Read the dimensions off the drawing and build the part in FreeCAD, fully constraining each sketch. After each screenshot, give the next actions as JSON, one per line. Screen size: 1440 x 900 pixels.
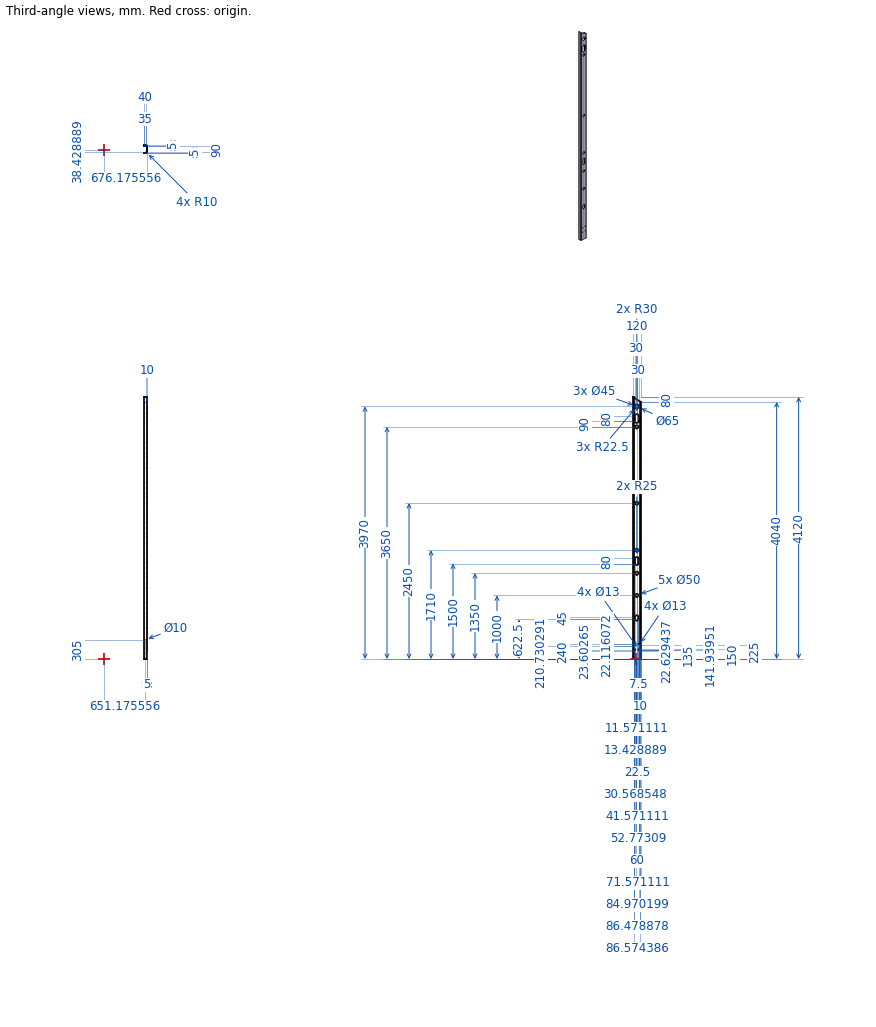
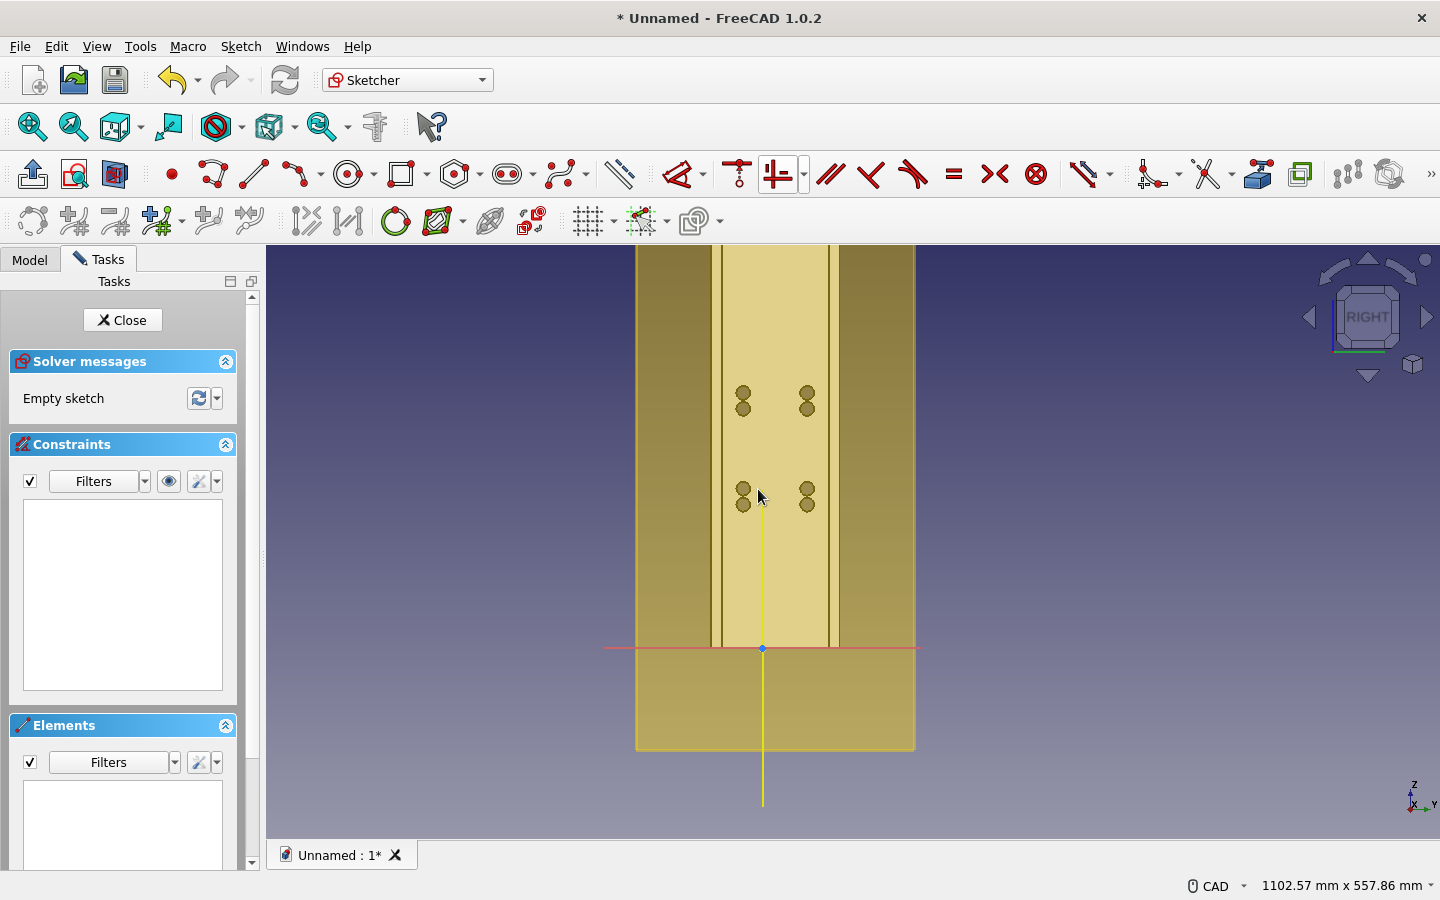
{"action": "key", "text": "g m"}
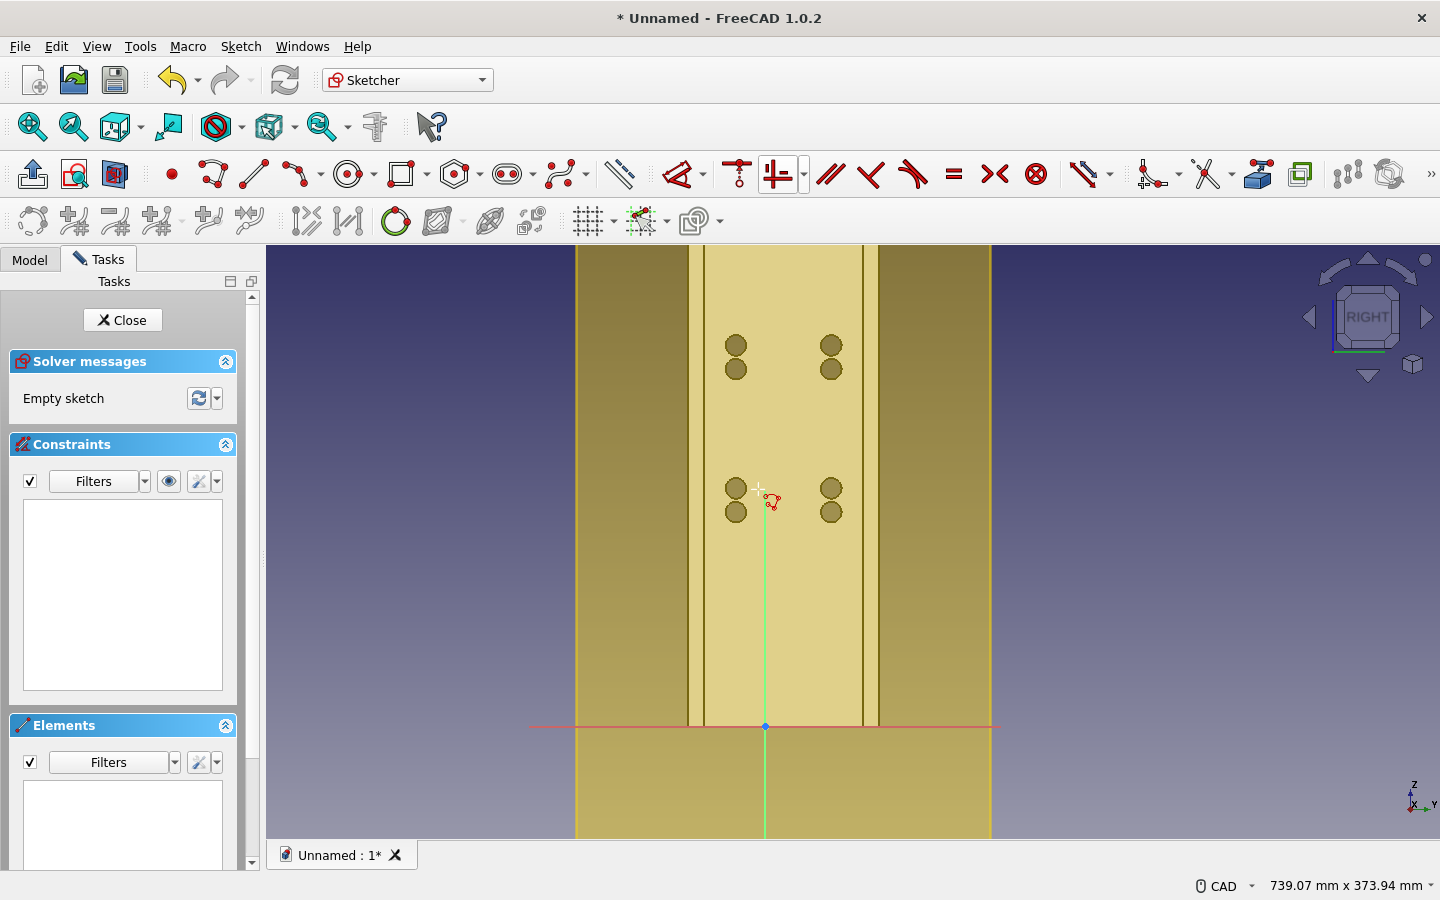
{"action": "left_click", "coordinate": [714, 392]}
{"action": "left_click", "coordinate": [851, 392]}
{"action": "left_click", "coordinate": [848, 357]}
{"action": "left_click", "coordinate": [714, 357]}
{"action": "left_click", "coordinate": [714, 393]}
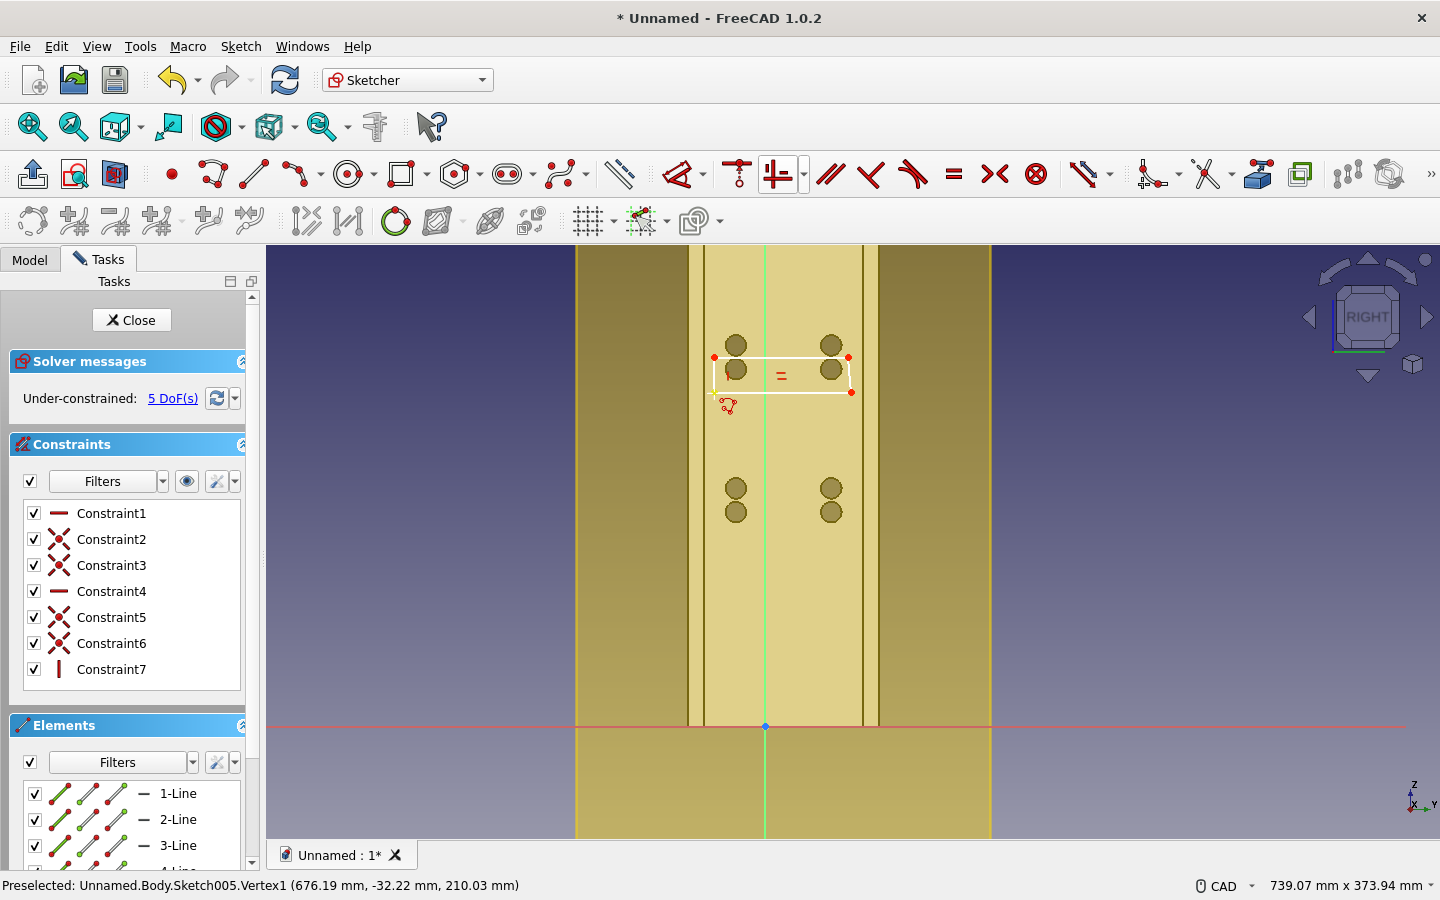
{"action": "left_click", "coordinate": [717, 537]}
{"action": "left_click", "coordinate": [854, 537]}
{"action": "left_click", "coordinate": [854, 501]}
{"action": "left_click", "coordinate": [717, 493]}
{"action": "left_click", "coordinate": [717, 538]}
{"action": "key", "text": "Escape"}
{"action": "key", "text": "Escape"}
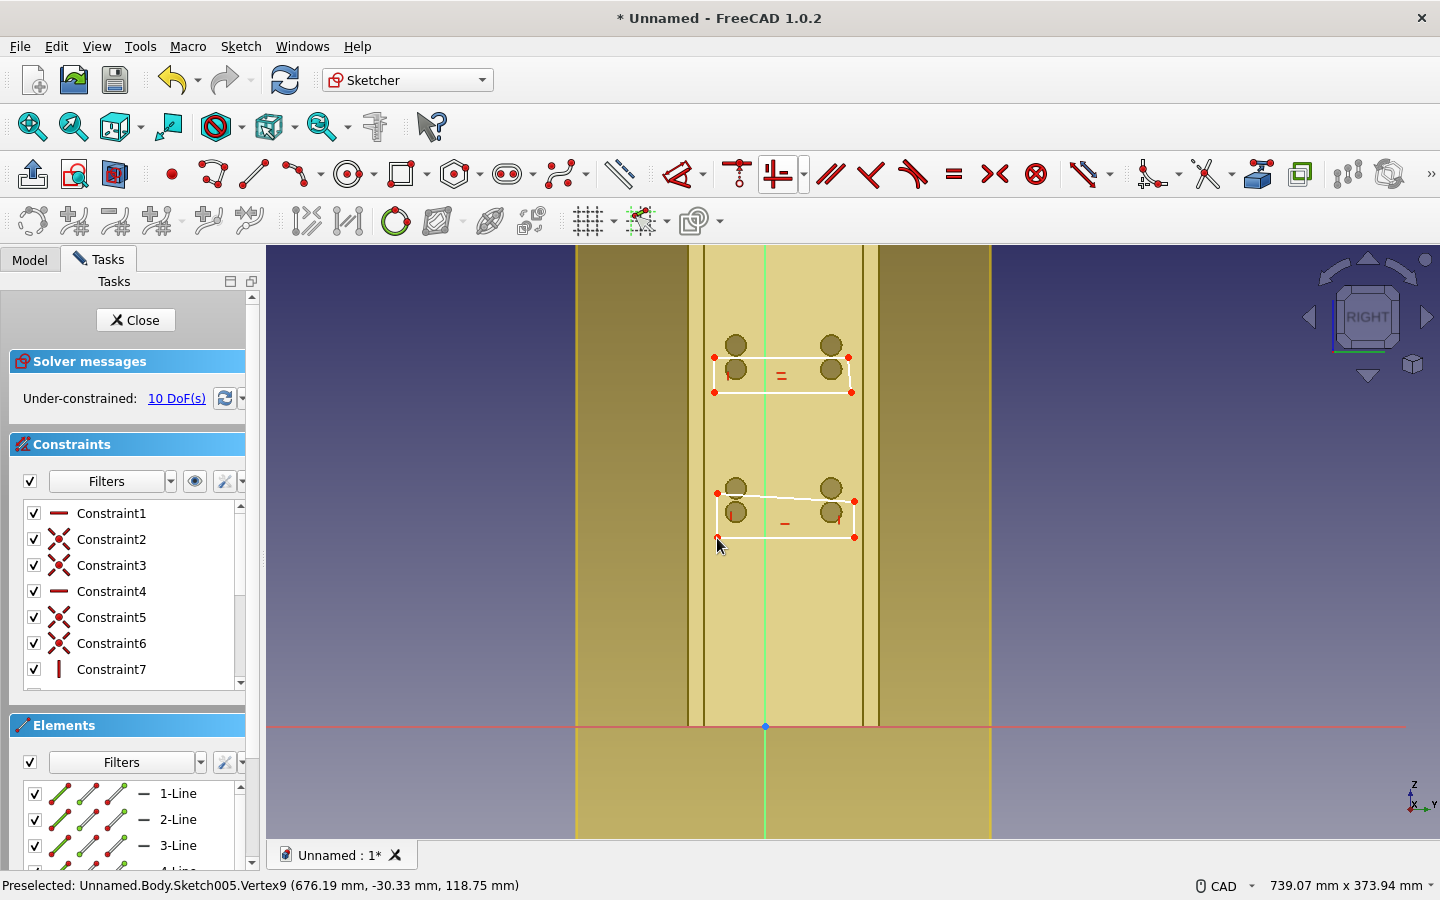
{"action": "left_click", "coordinate": [676, 174]}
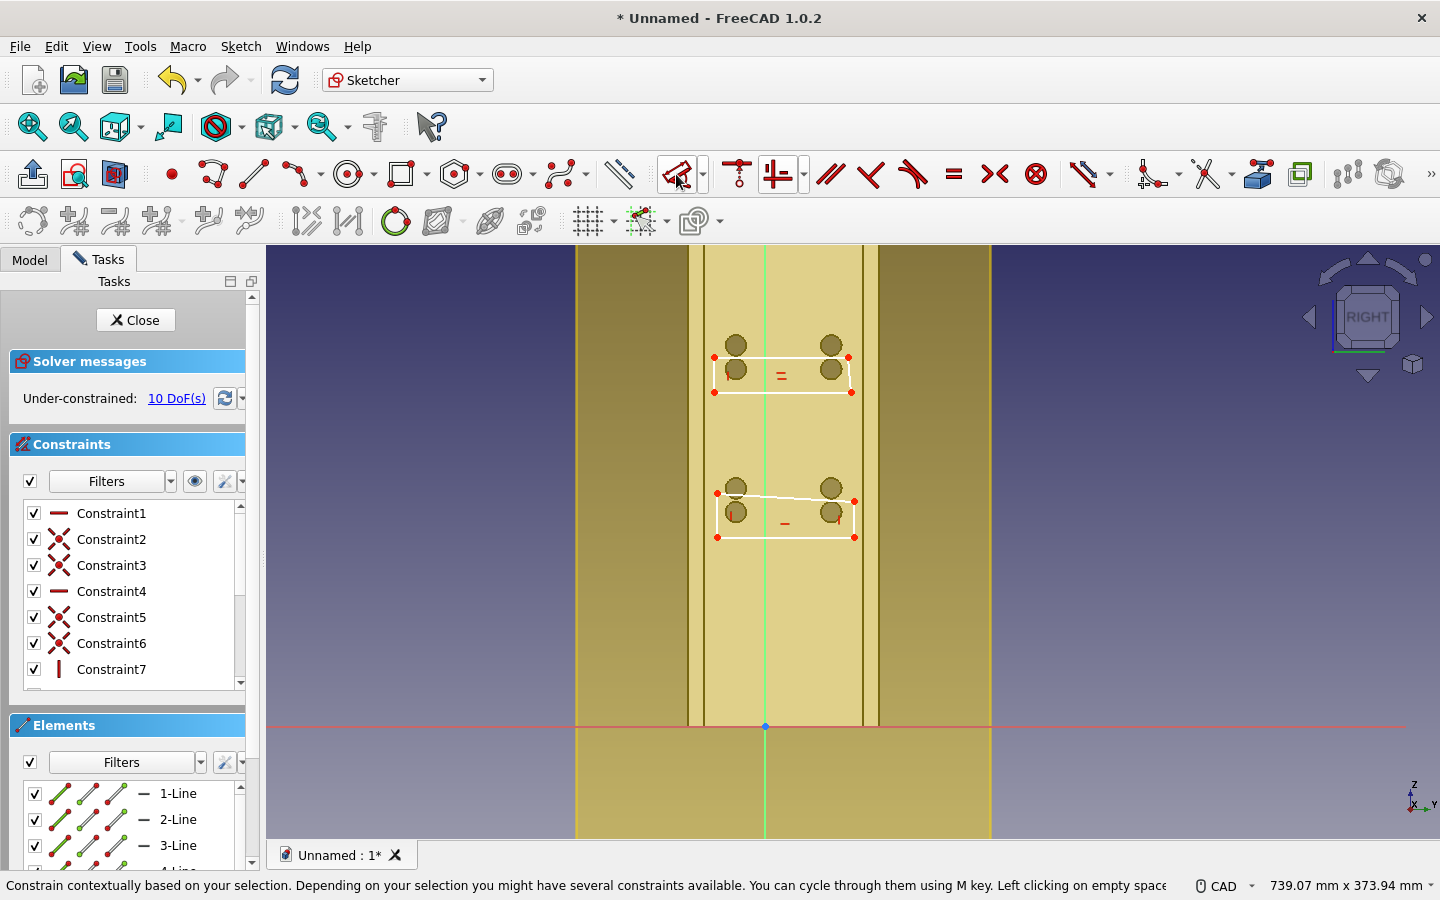
{"action": "left_click", "coordinate": [717, 507]}
{"action": "left_click", "coordinate": [683, 516]}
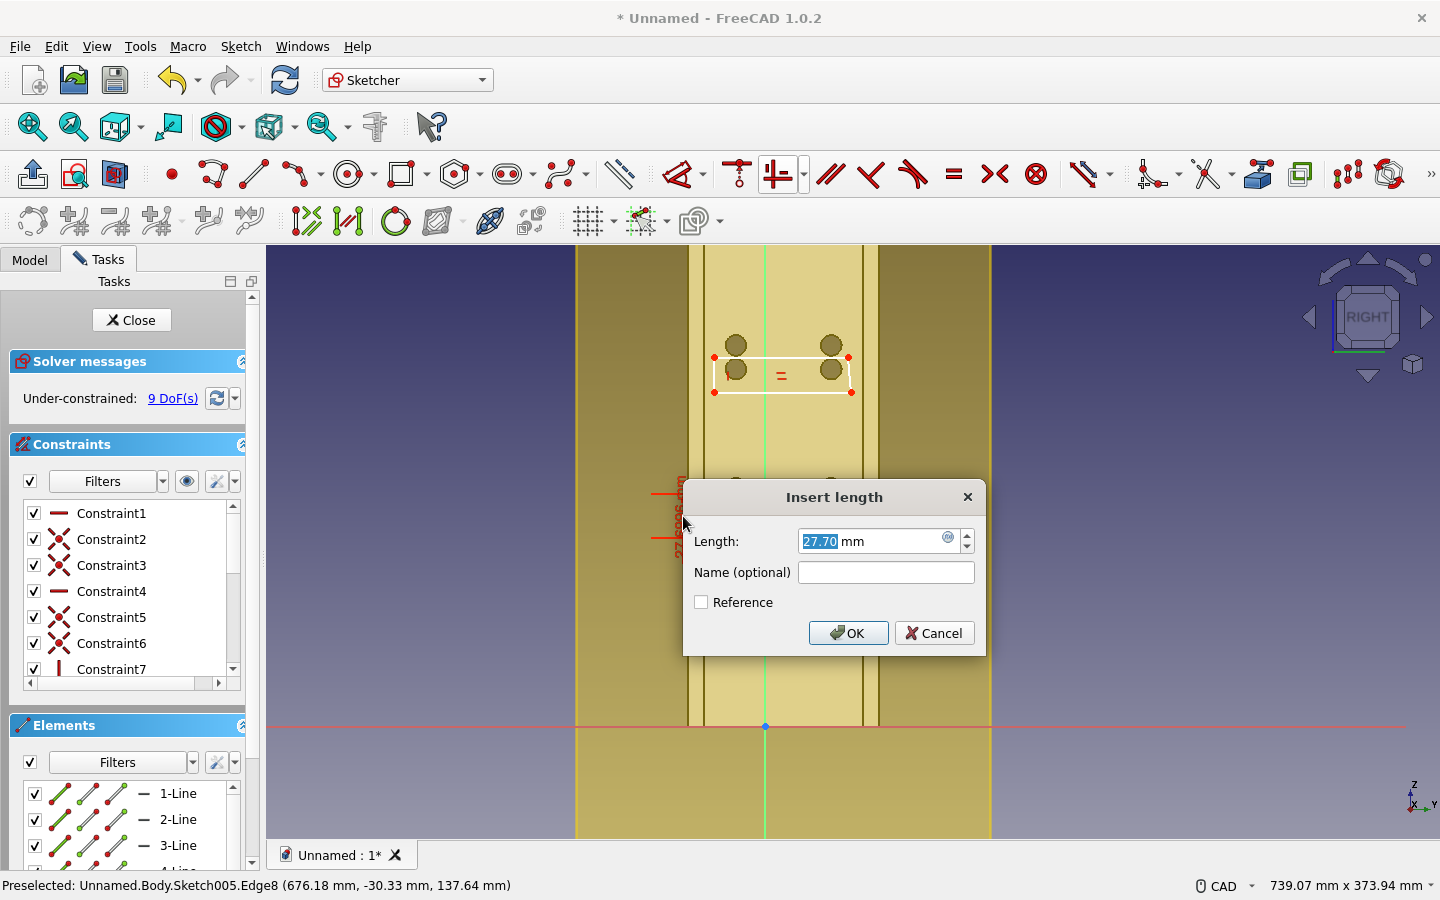
{"action": "type", "text": "23.60265"}
{"action": "key", "text": "Return"}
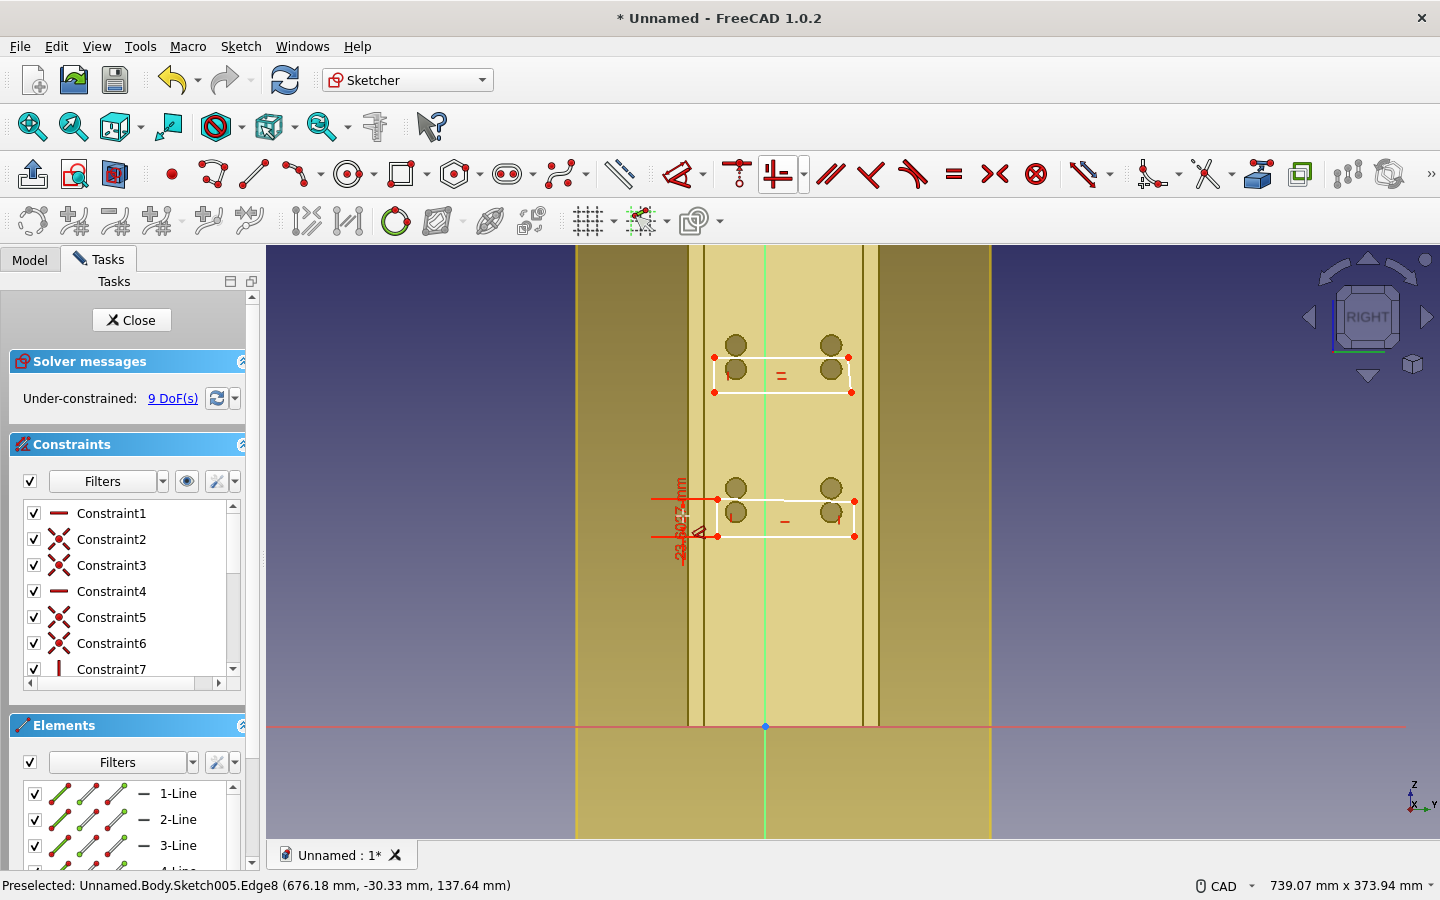
{"action": "scroll", "coordinate": [755, 393], "scroll_direction": "up", "scroll_amount": 2}